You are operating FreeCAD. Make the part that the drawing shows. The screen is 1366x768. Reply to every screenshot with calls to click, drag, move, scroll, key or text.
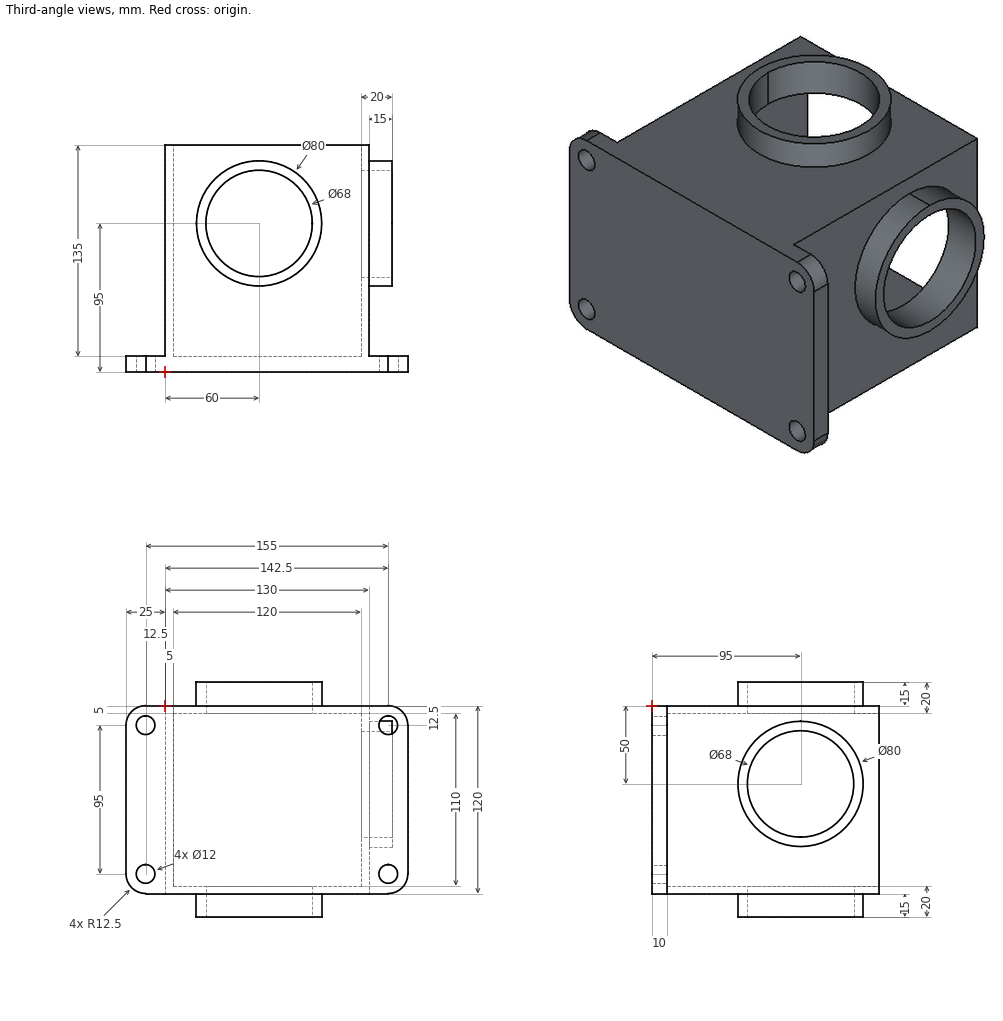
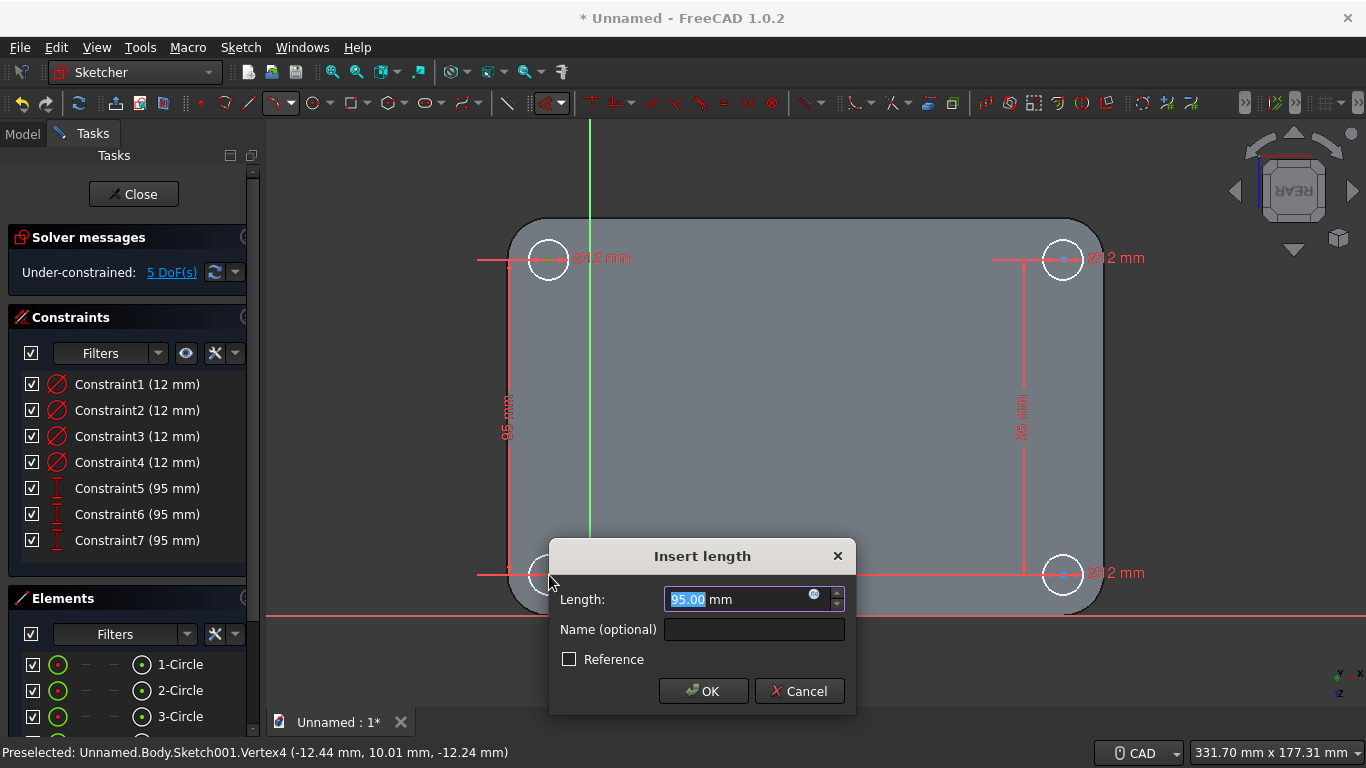
text(95)
key(Return)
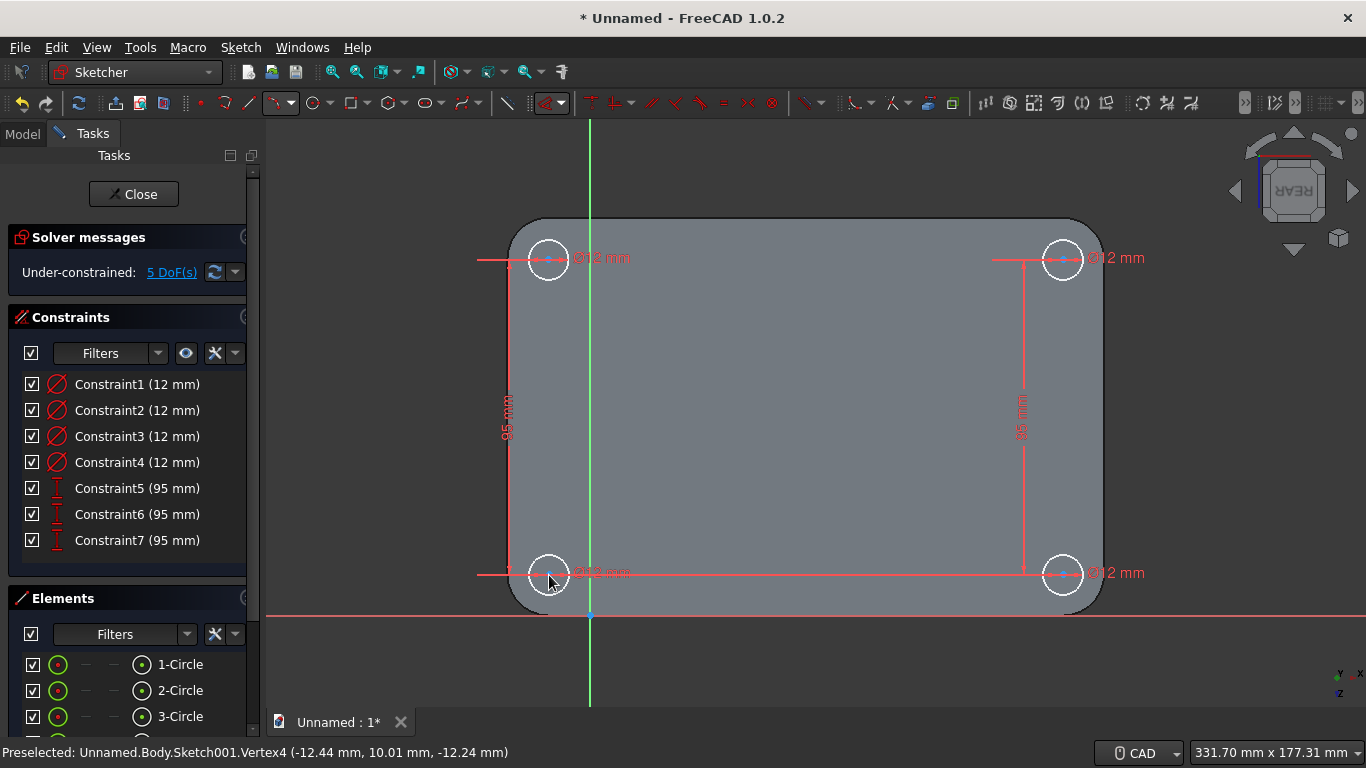
click(549, 260)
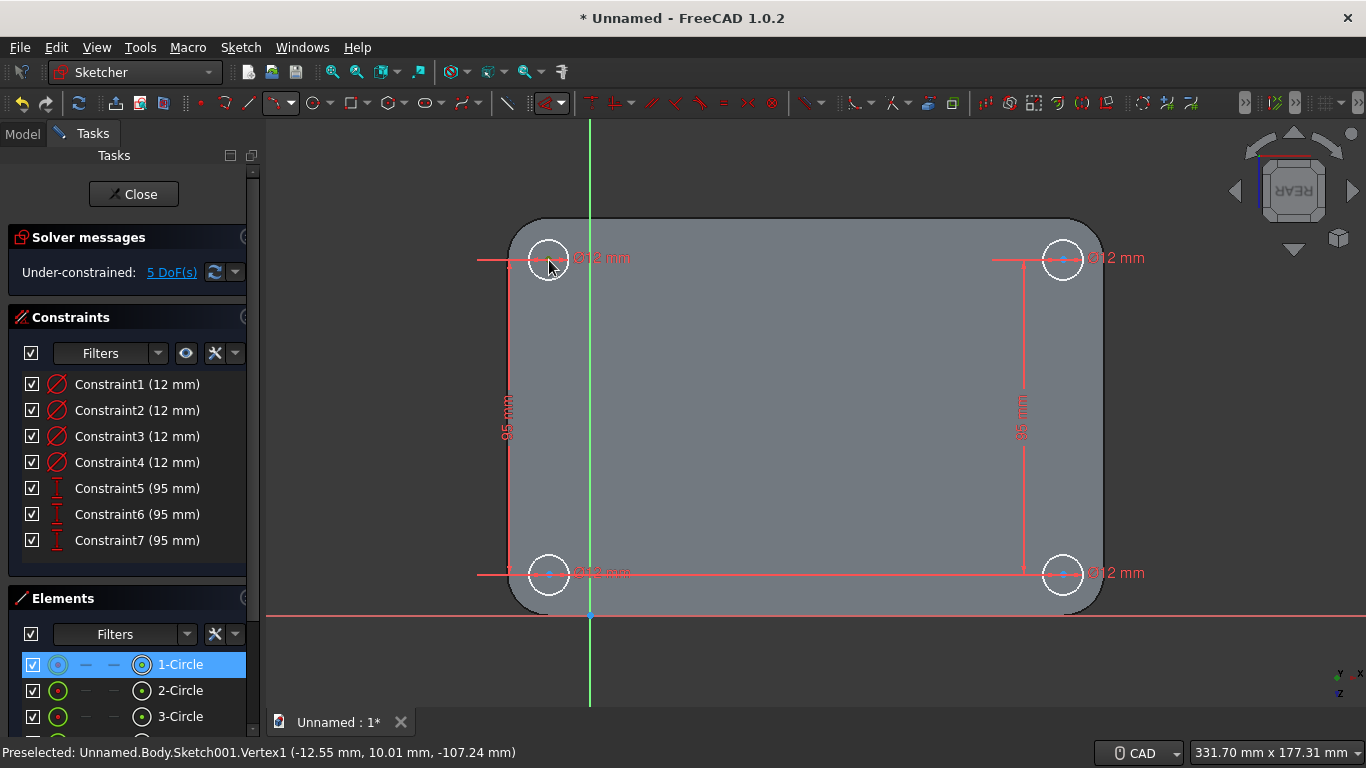
key(l)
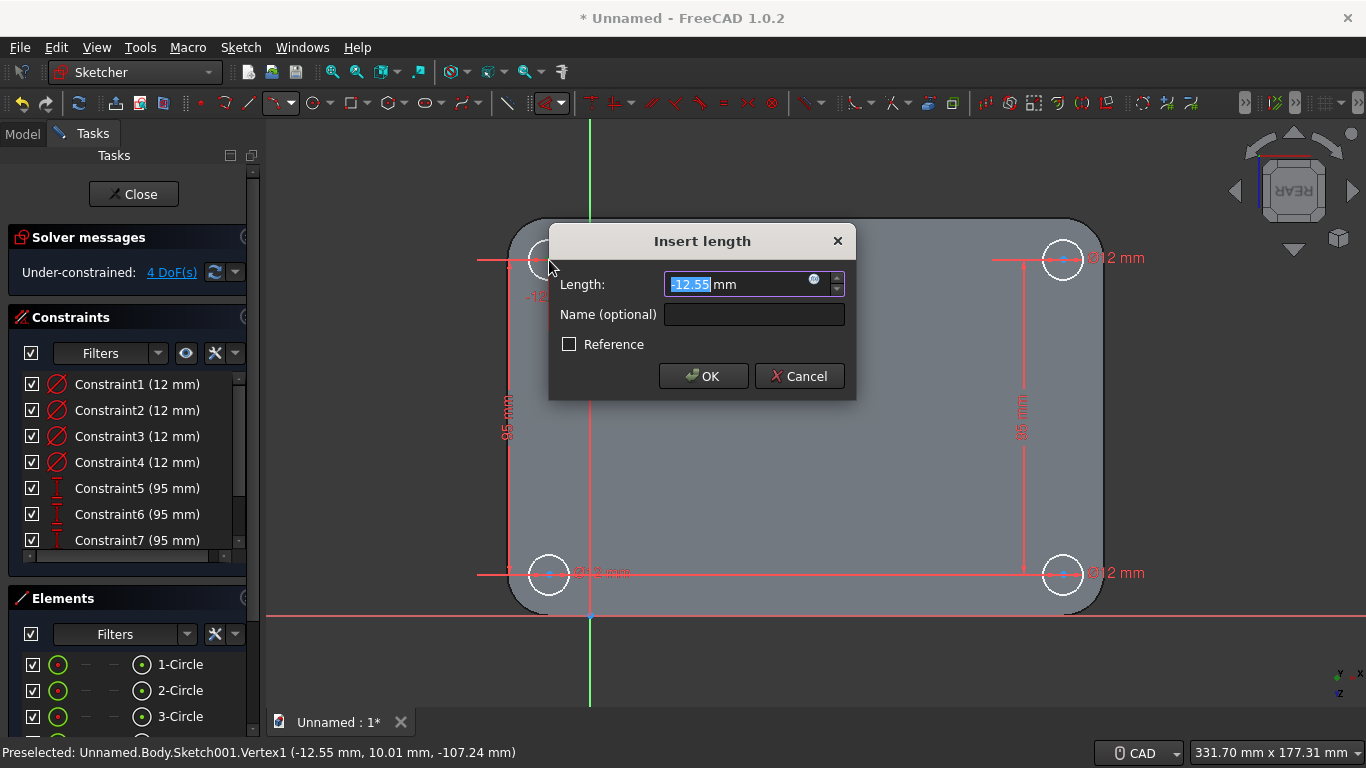
text(-12.5)
key(Return)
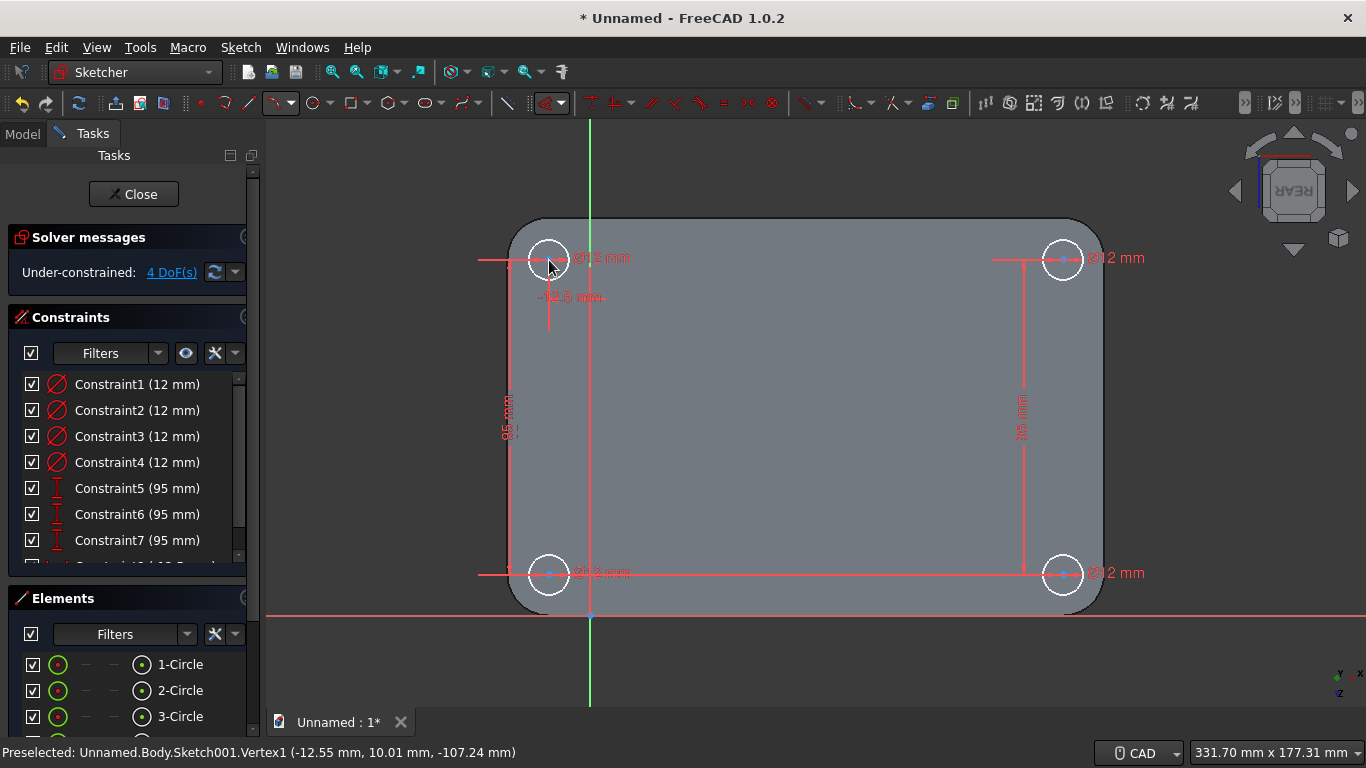
click(1063, 575)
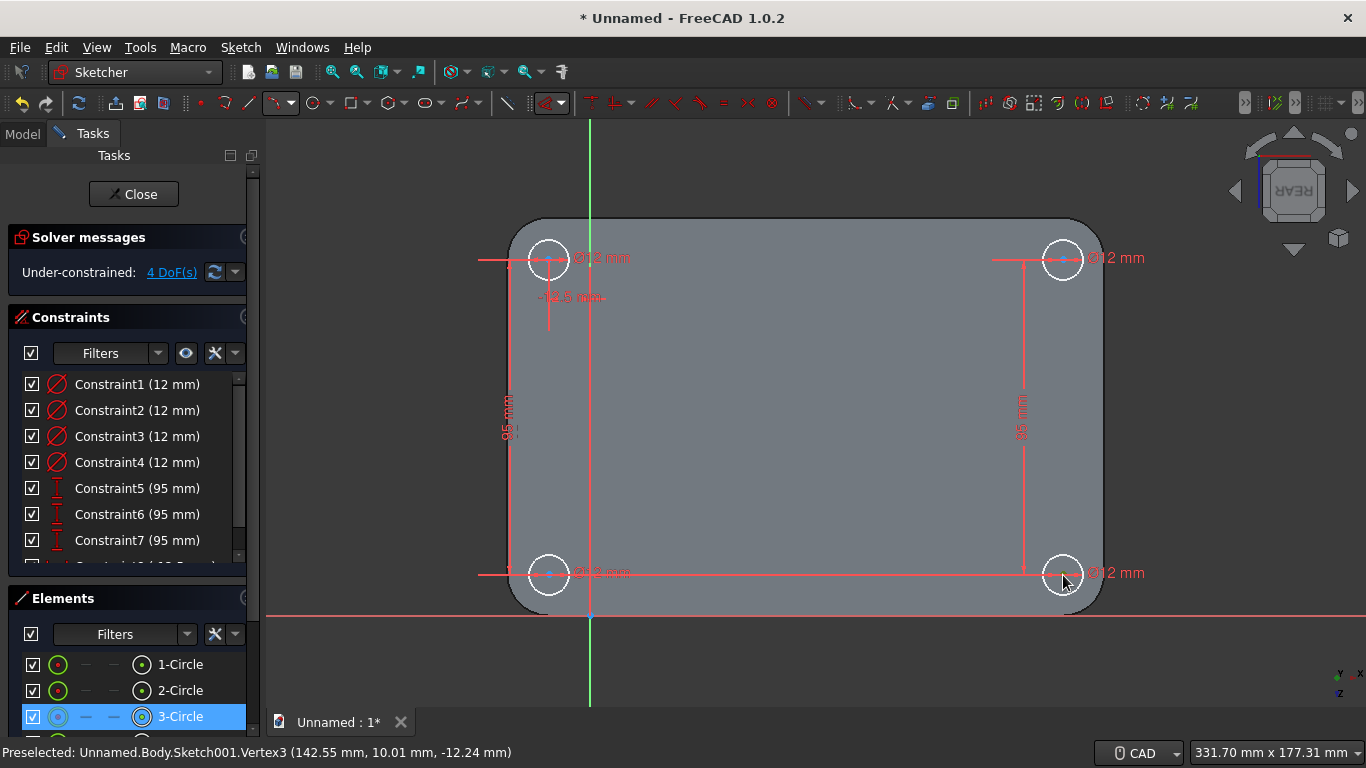
key(i)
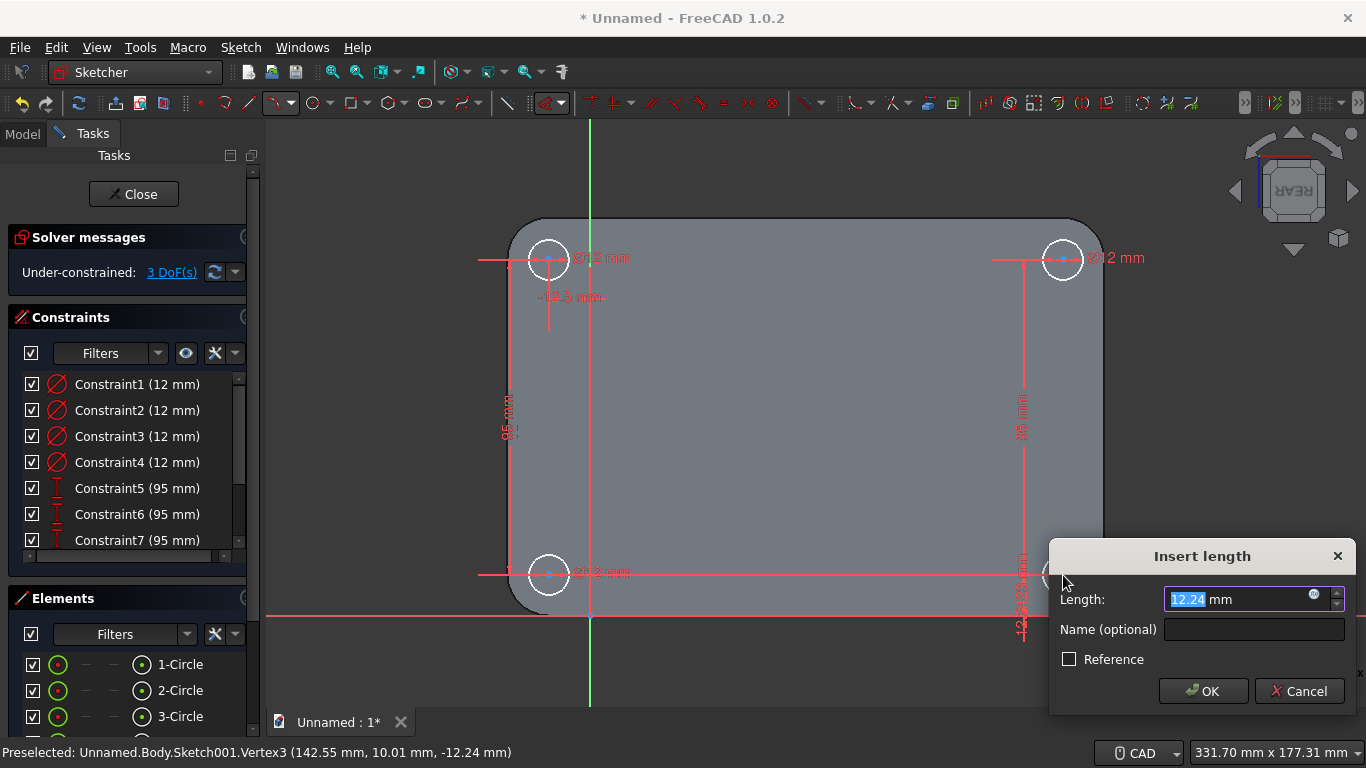
text(12.5)
key(Return)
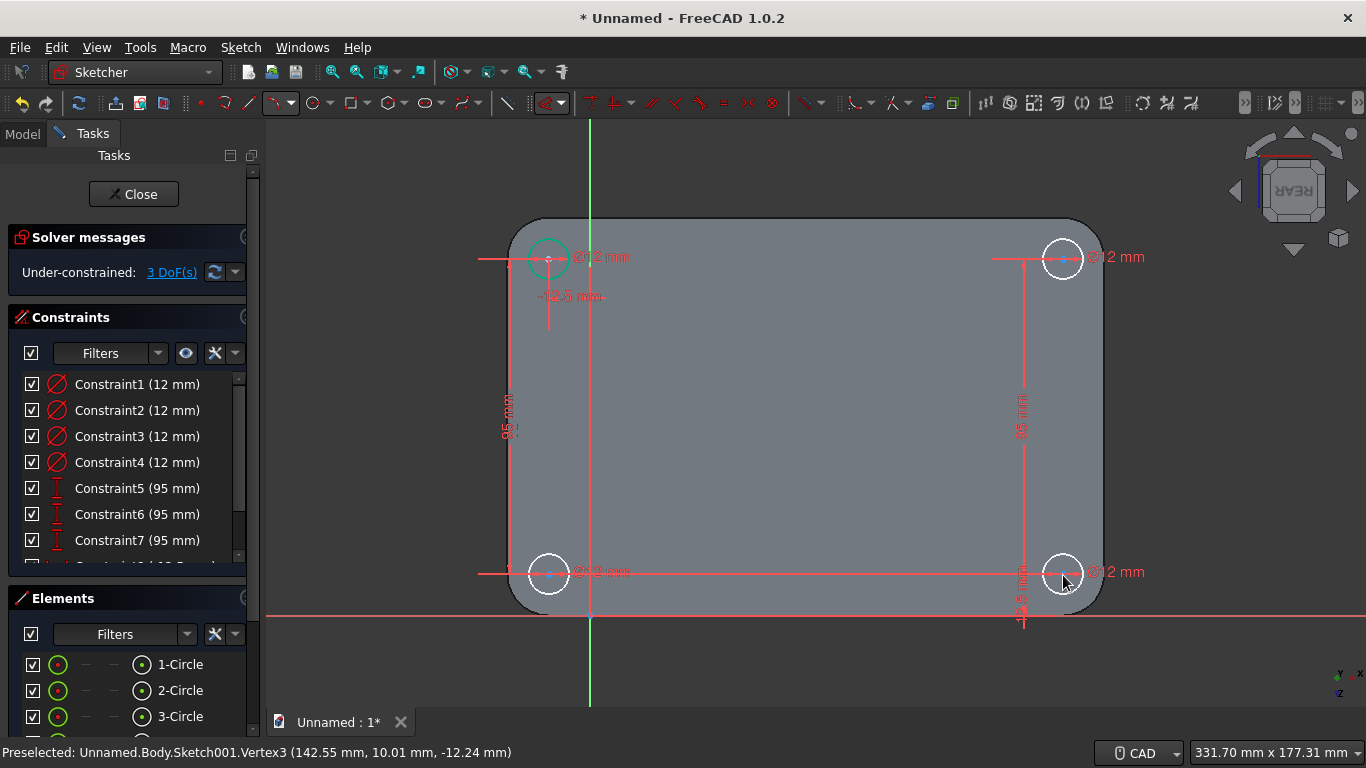
click(549, 574)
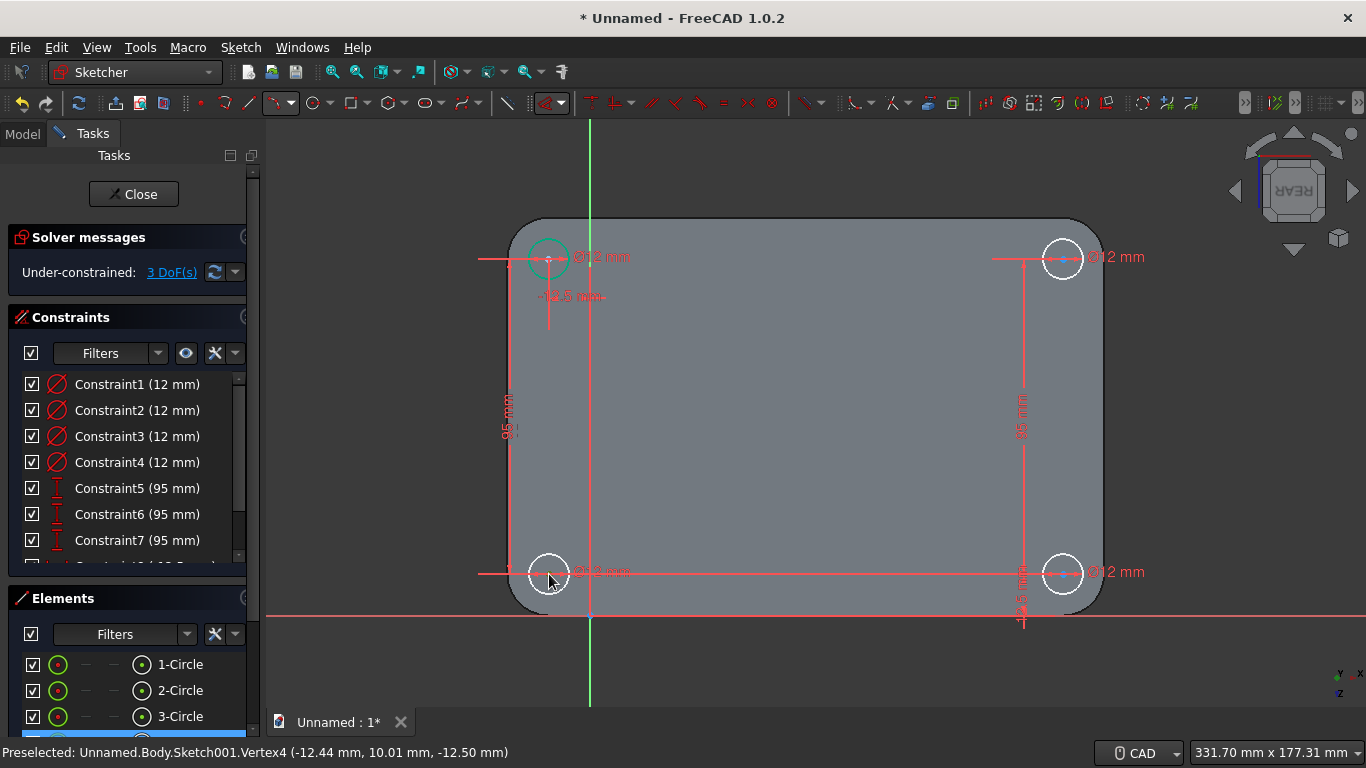
key(l)